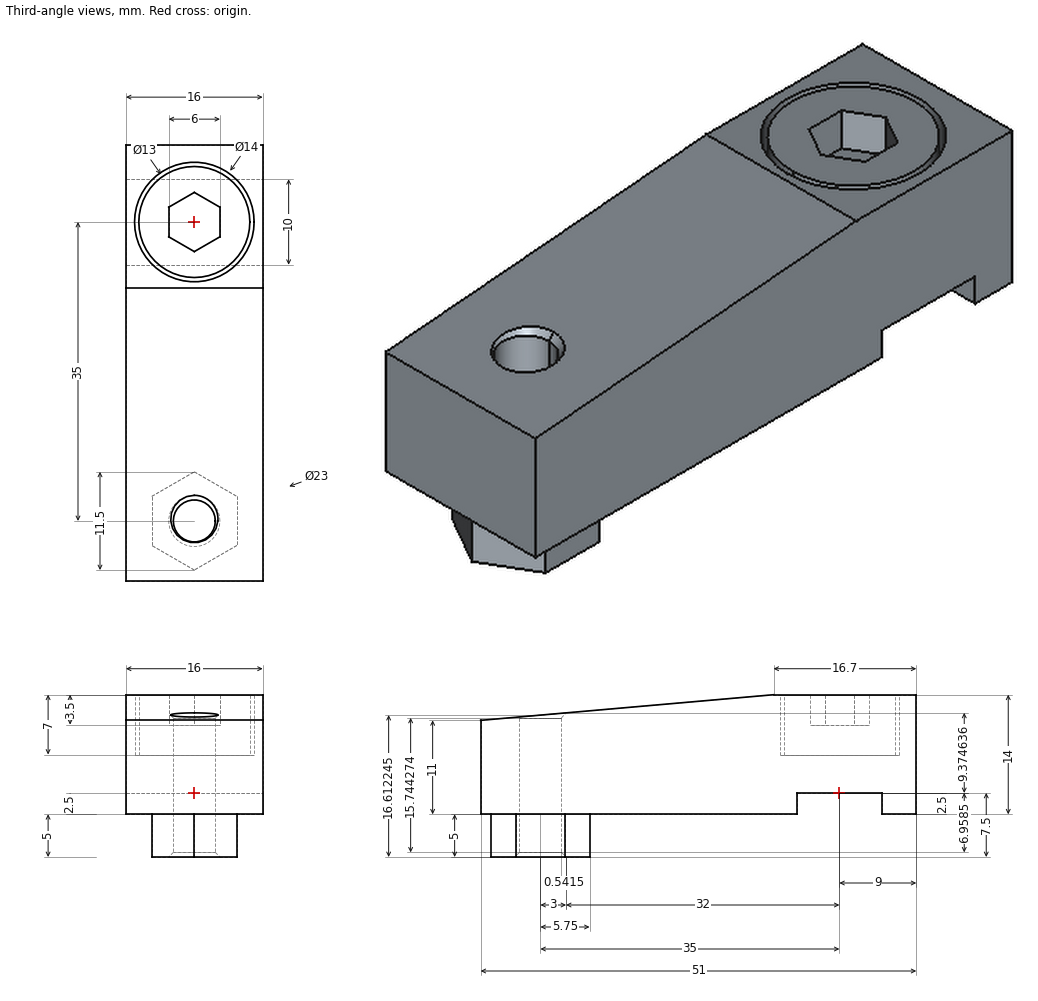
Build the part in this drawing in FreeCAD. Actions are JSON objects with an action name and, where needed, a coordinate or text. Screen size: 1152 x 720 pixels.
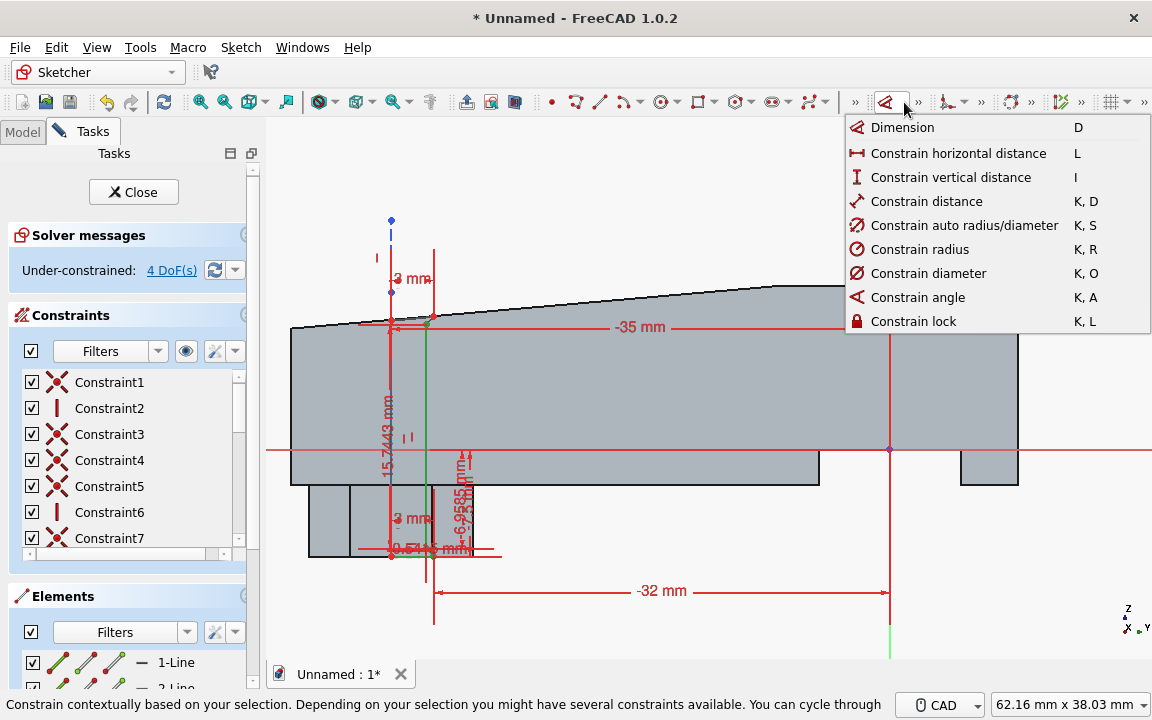
{"action": "left_click", "coordinate": [998, 177]}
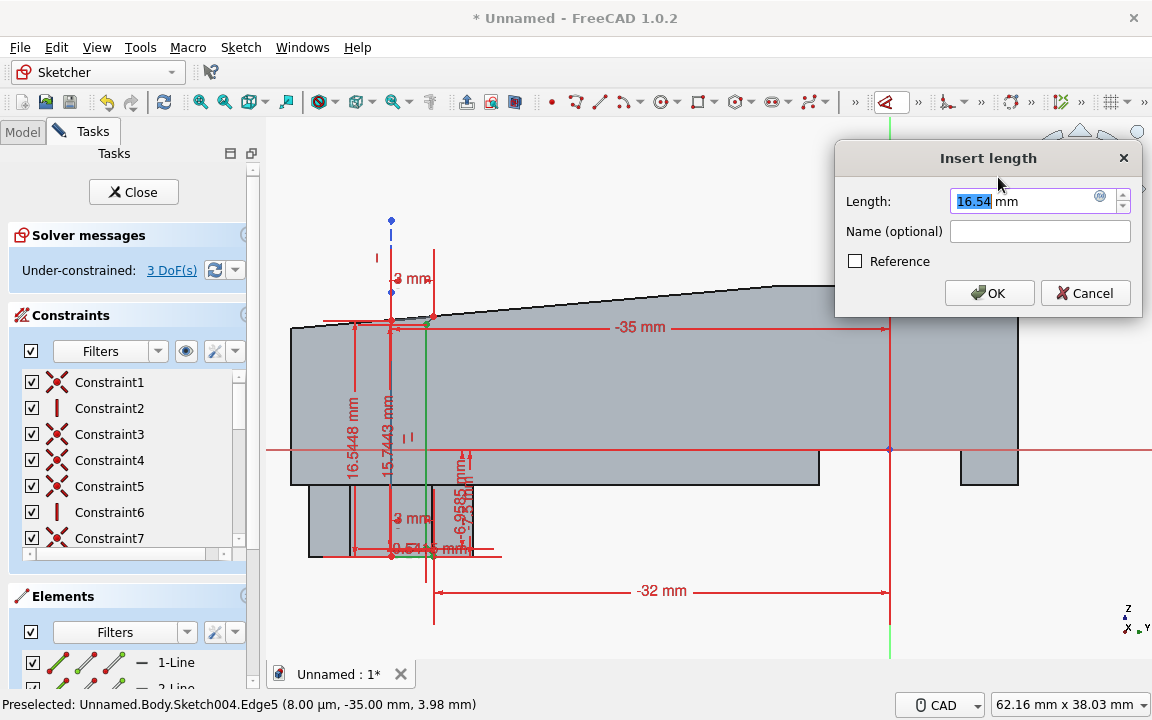
{"action": "type", "text": "16.612245"}
{"action": "key", "text": "Return"}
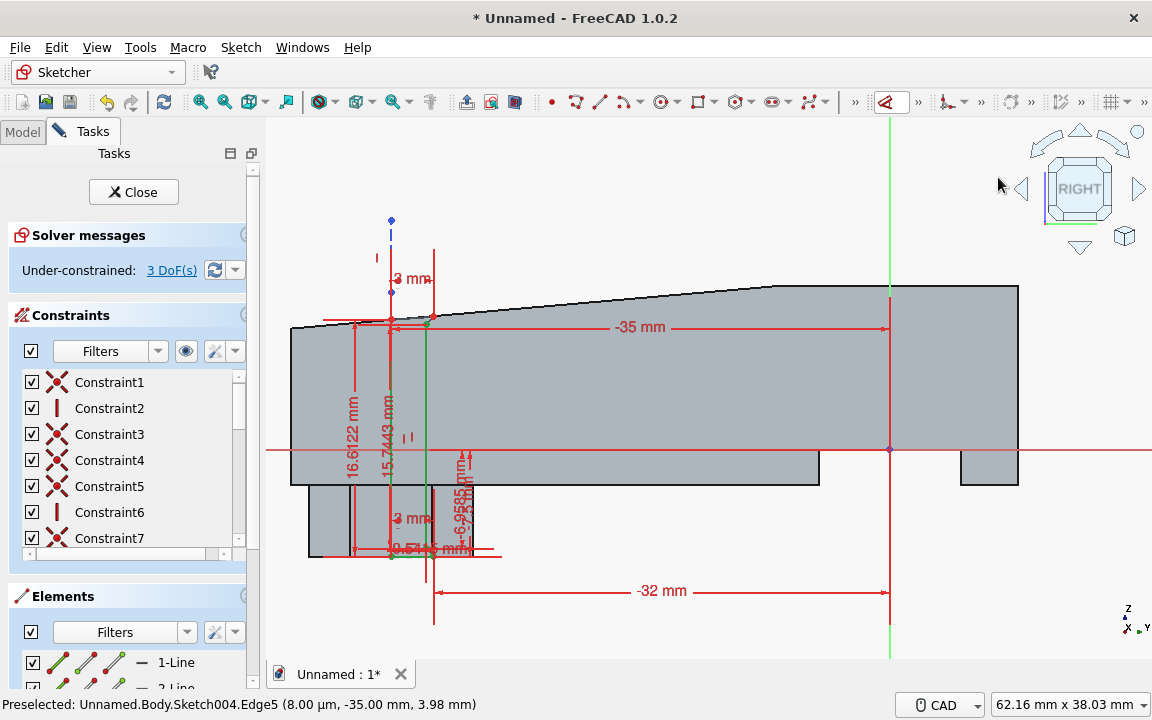
{"action": "left_click", "coordinate": [434, 317]}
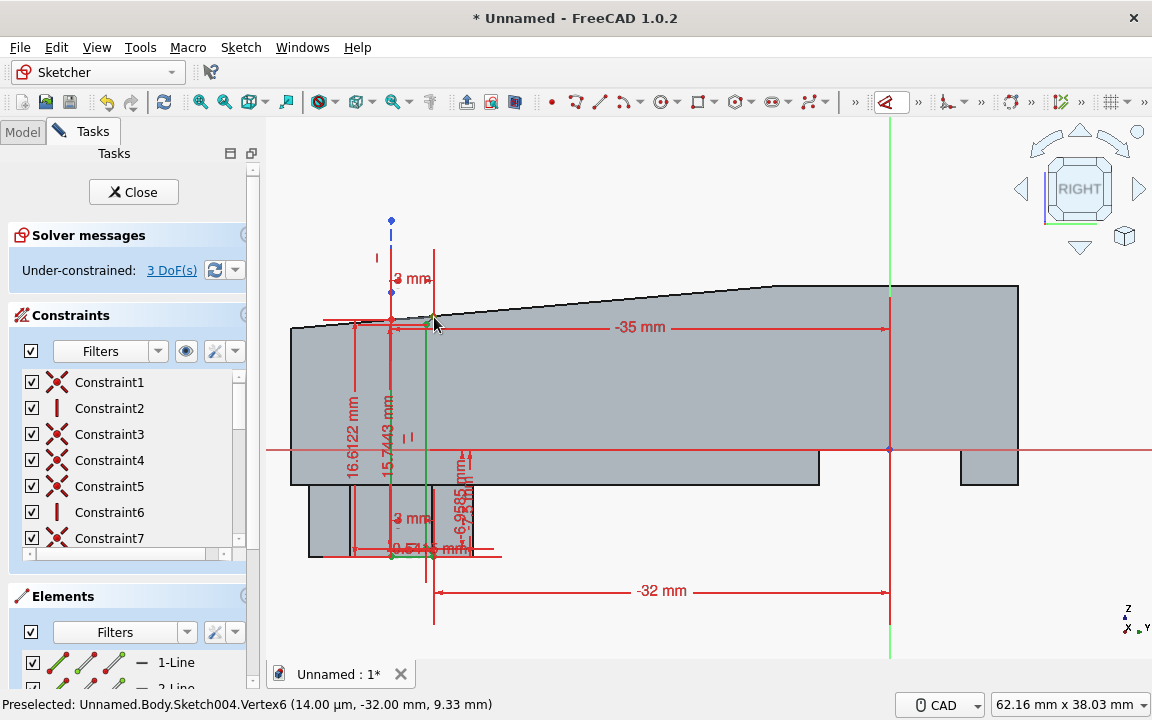
{"action": "key", "text": "i"}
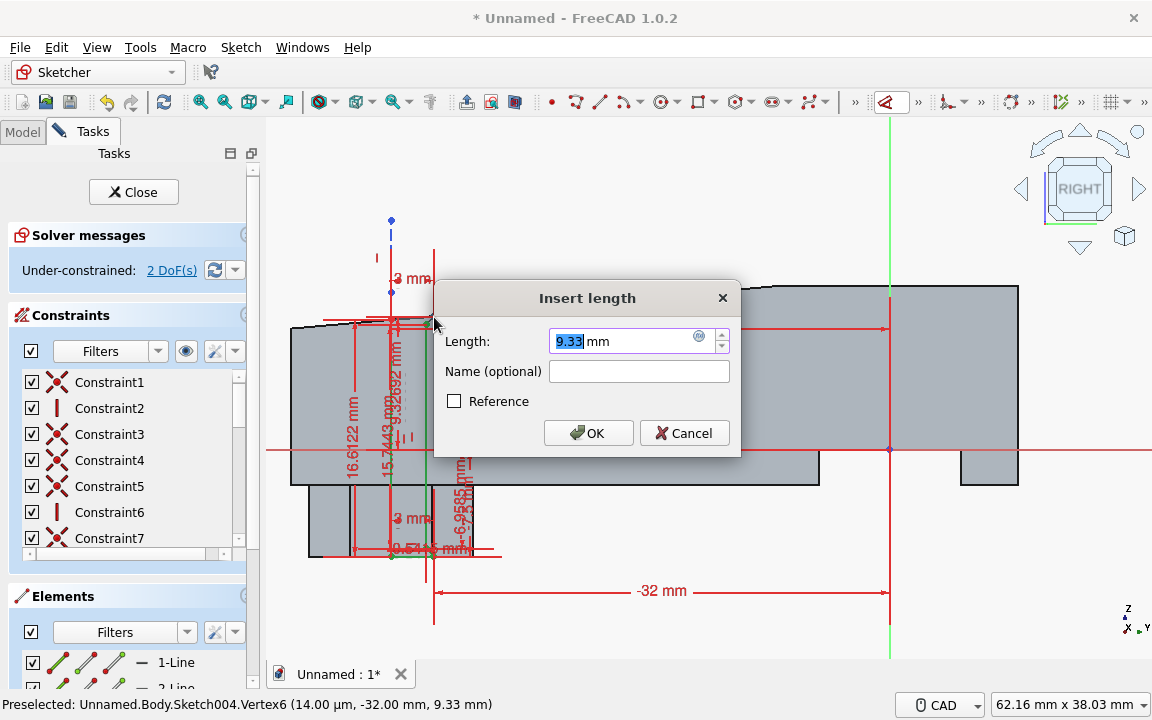
{"action": "type", "text": "9.374636"}
{"action": "key", "text": "Return"}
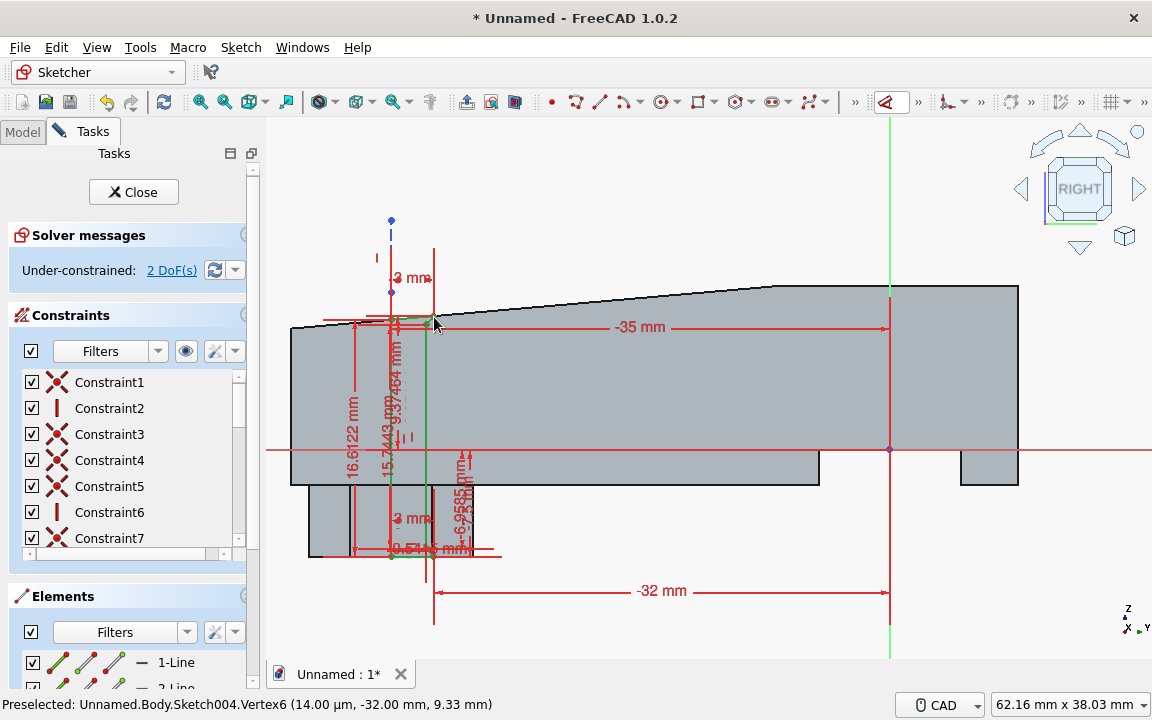
{"action": "left_click", "coordinate": [134, 192]}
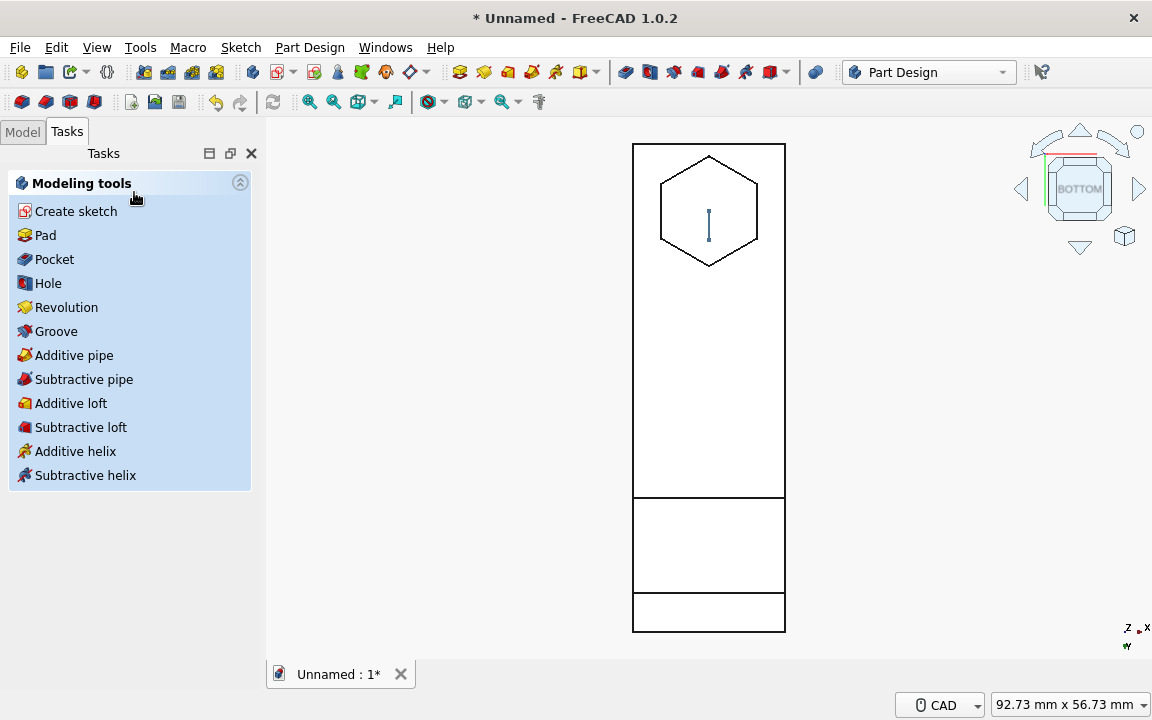
{"action": "left_click", "coordinate": [674, 72]}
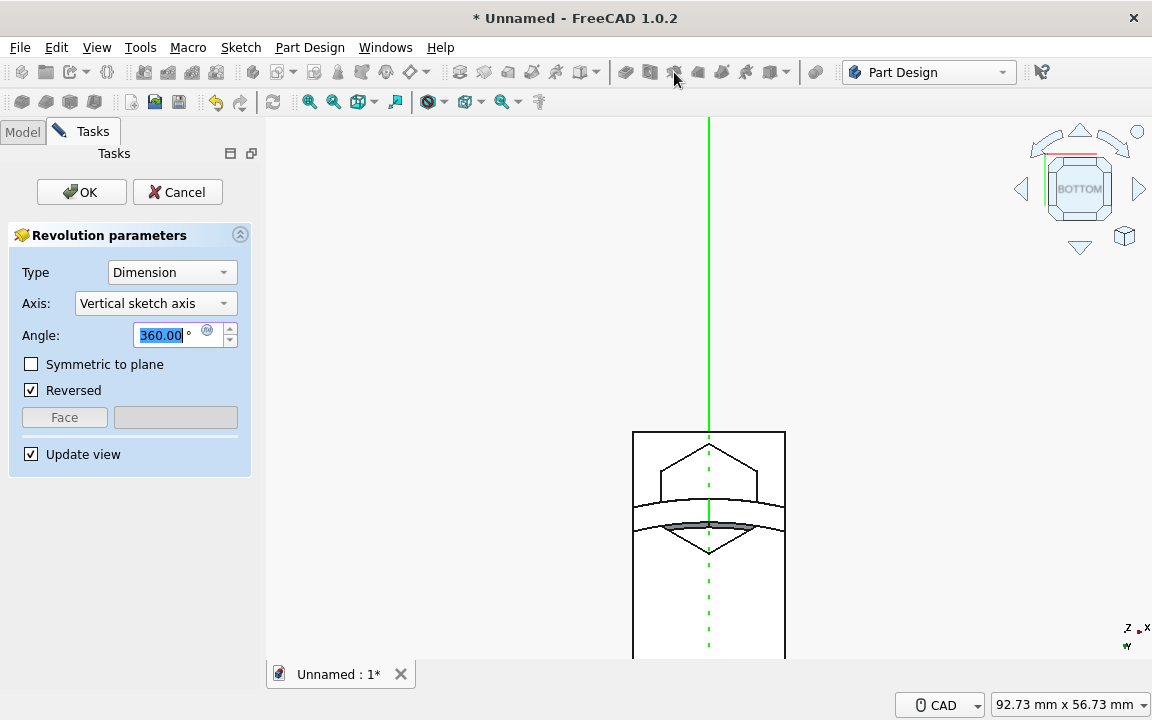
{"action": "left_click", "coordinate": [156, 304]}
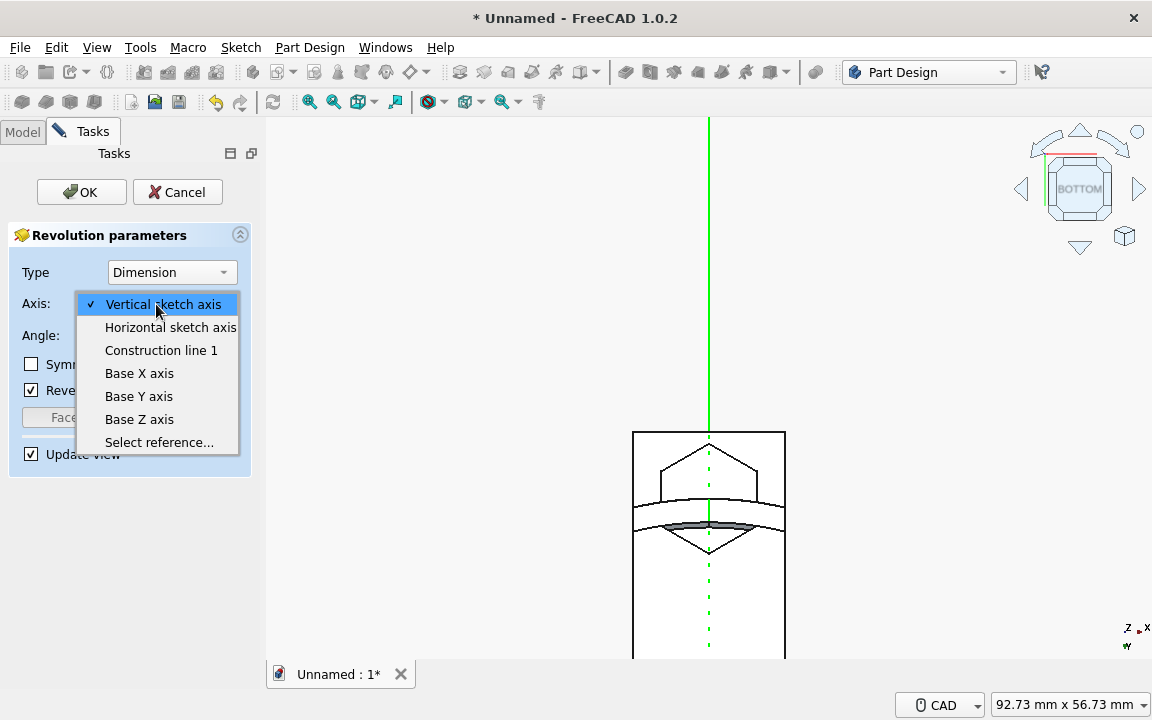
{"action": "left_click", "coordinate": [156, 350]}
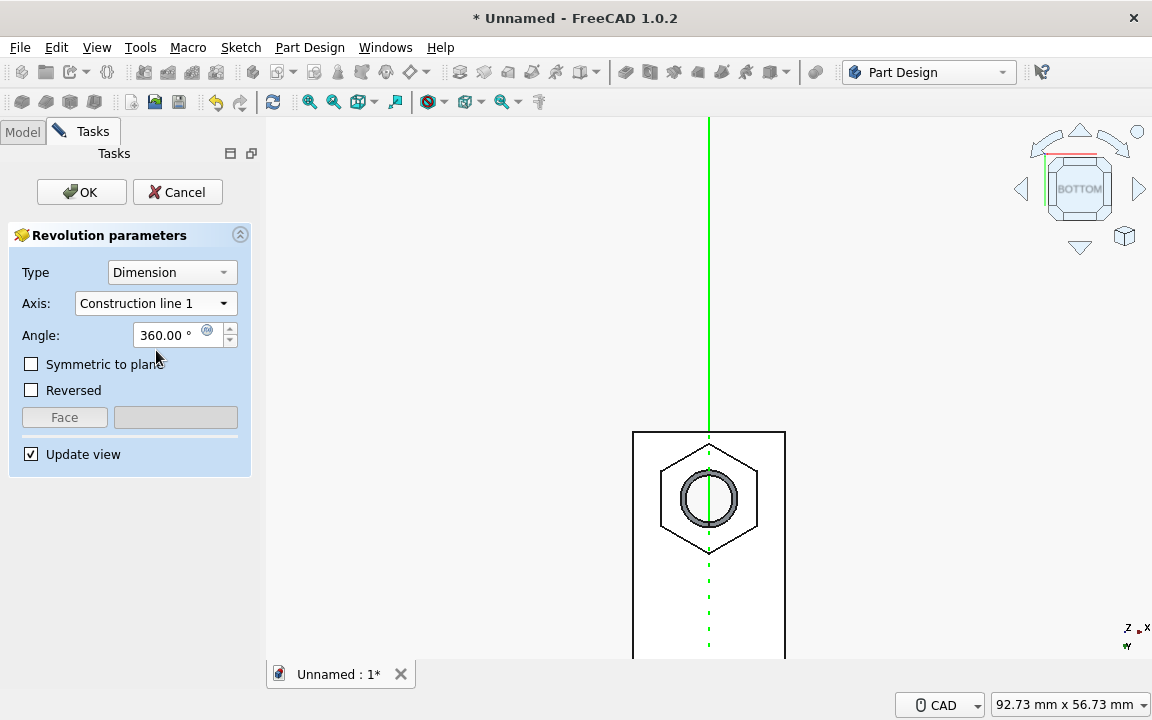
{"action": "left_click", "coordinate": [82, 192]}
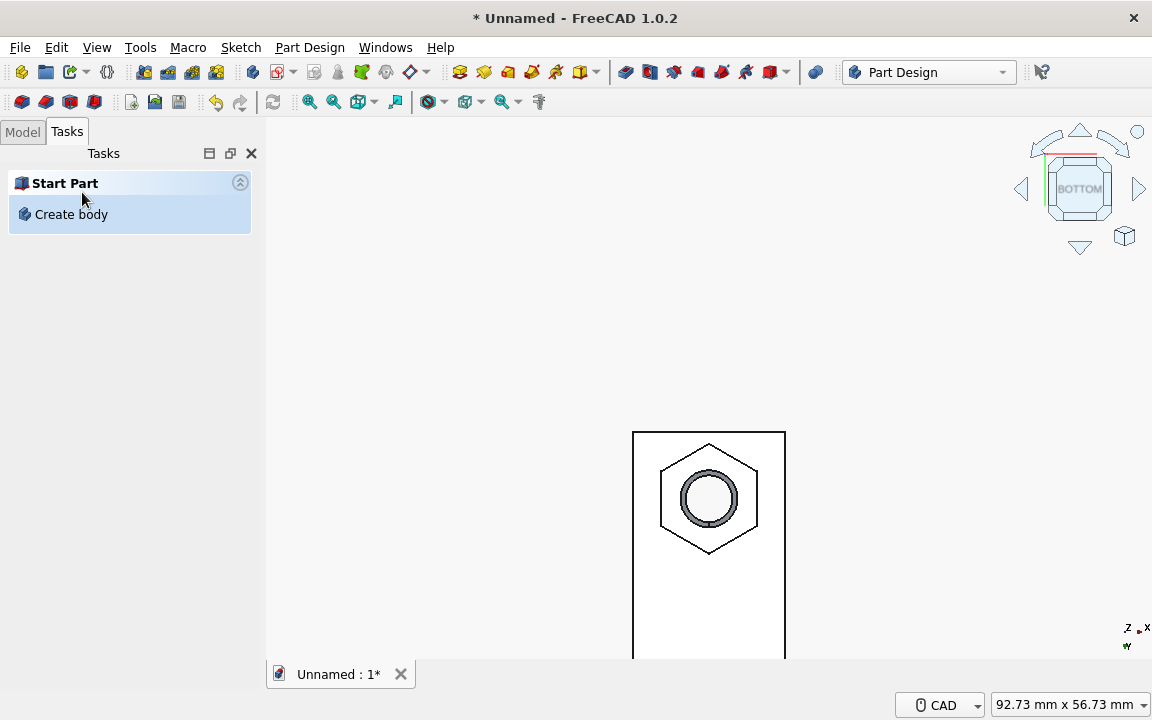
{"action": "key", "text": "v f"}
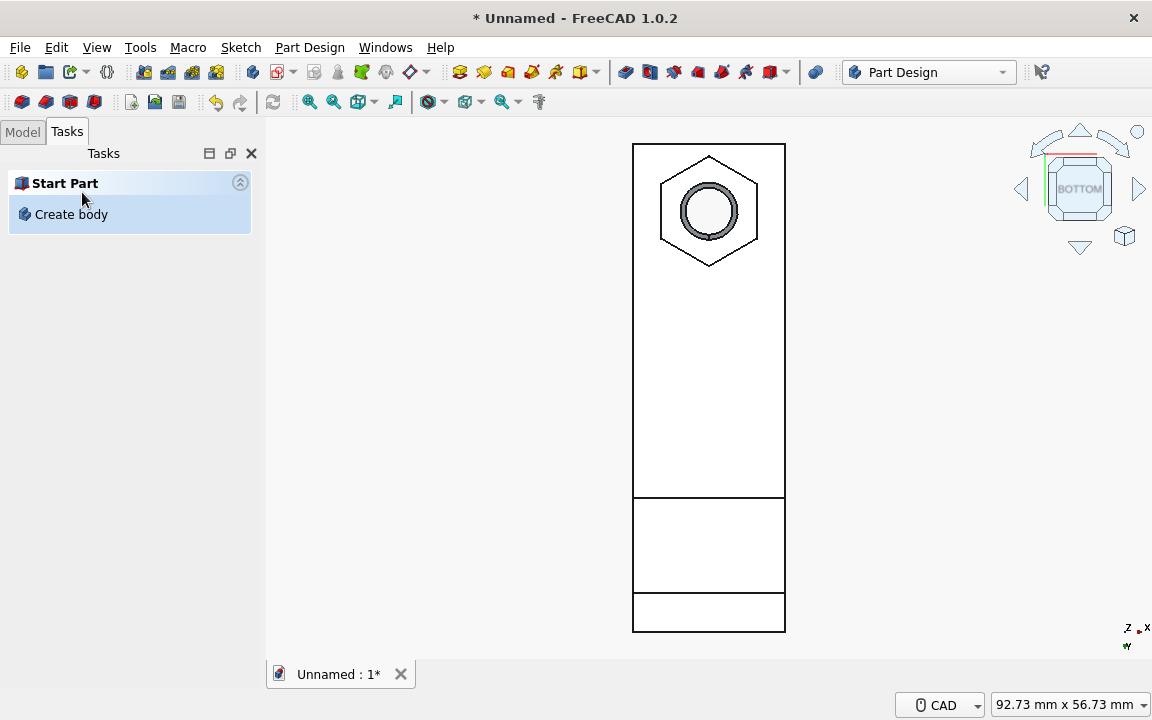
{"action": "key", "text": "0"}